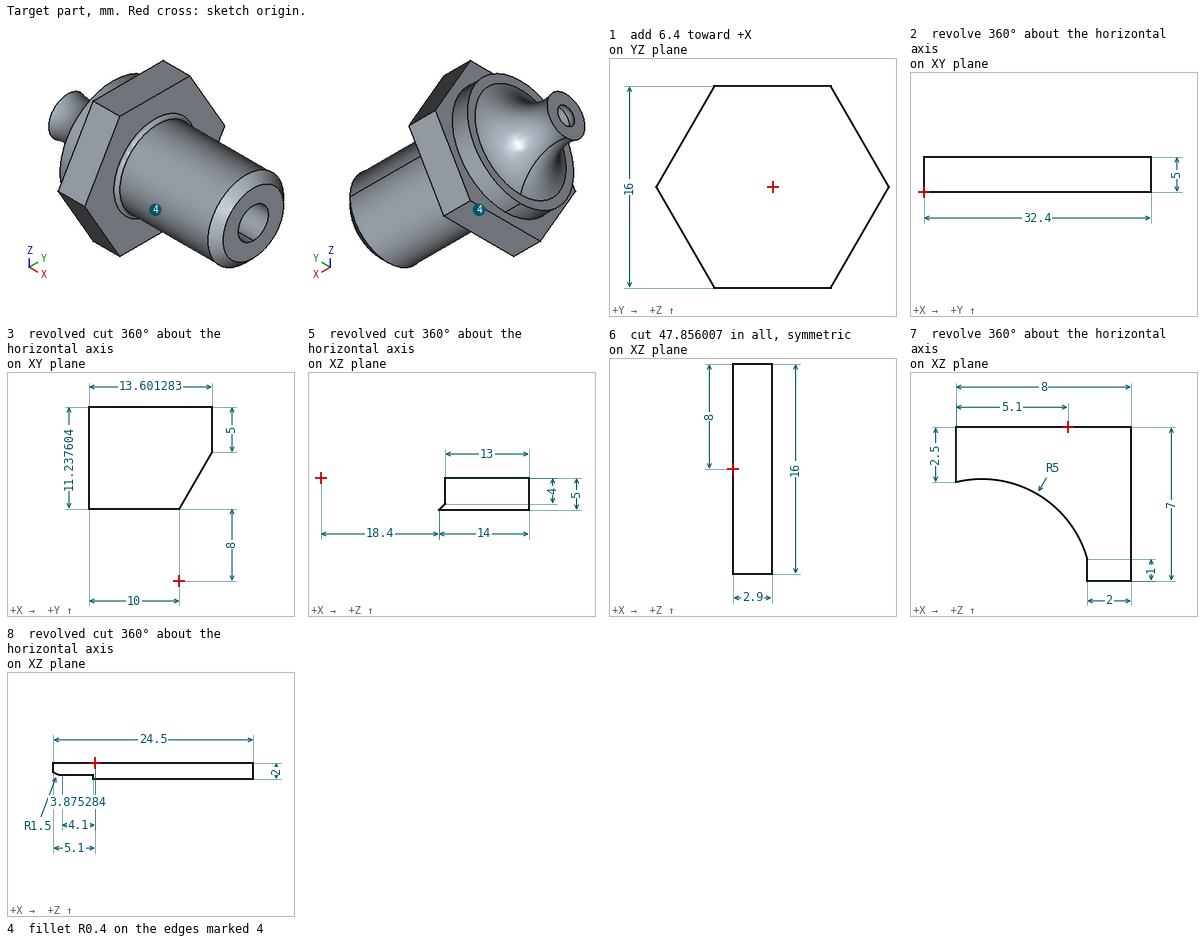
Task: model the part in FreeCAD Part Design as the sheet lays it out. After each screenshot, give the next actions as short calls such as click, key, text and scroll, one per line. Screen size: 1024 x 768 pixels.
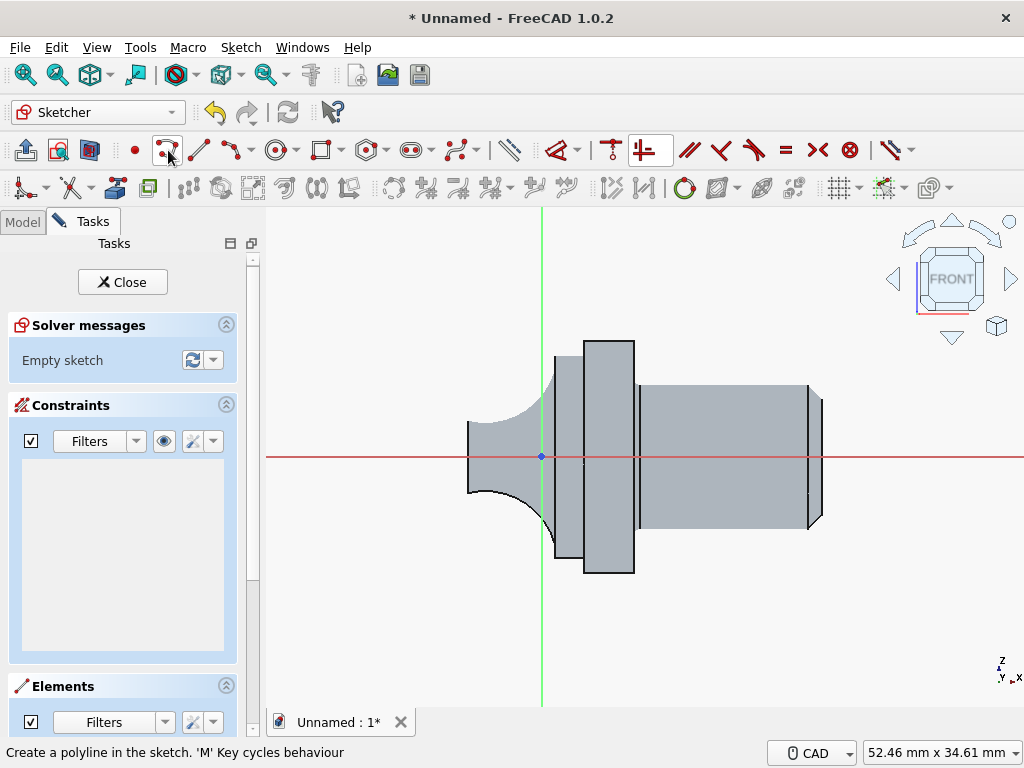
click(468, 473)
click(468, 457)
click(822, 466)
click(822, 486)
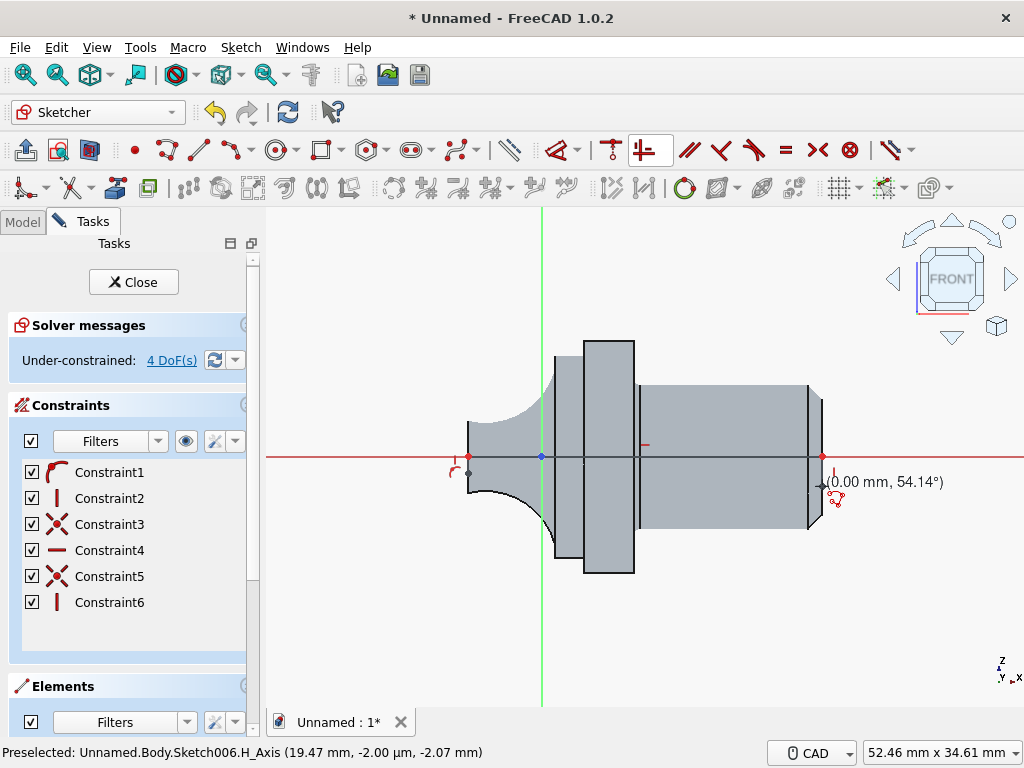
scroll(538, 486, up, 8)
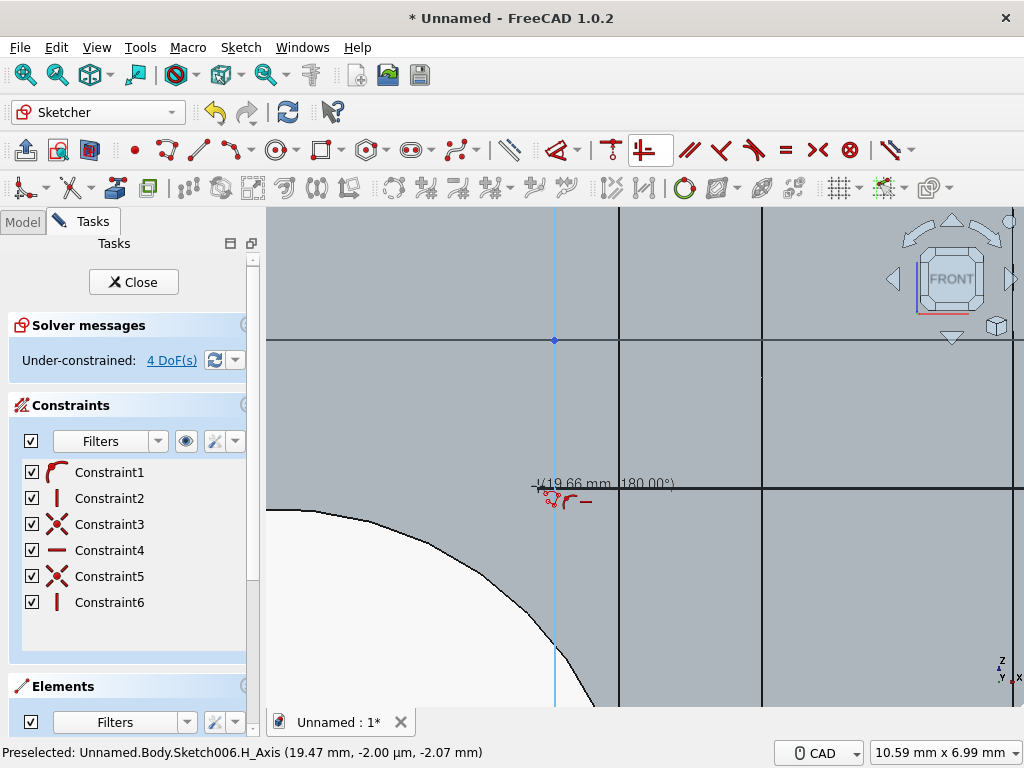
click(539, 484)
click(539, 447)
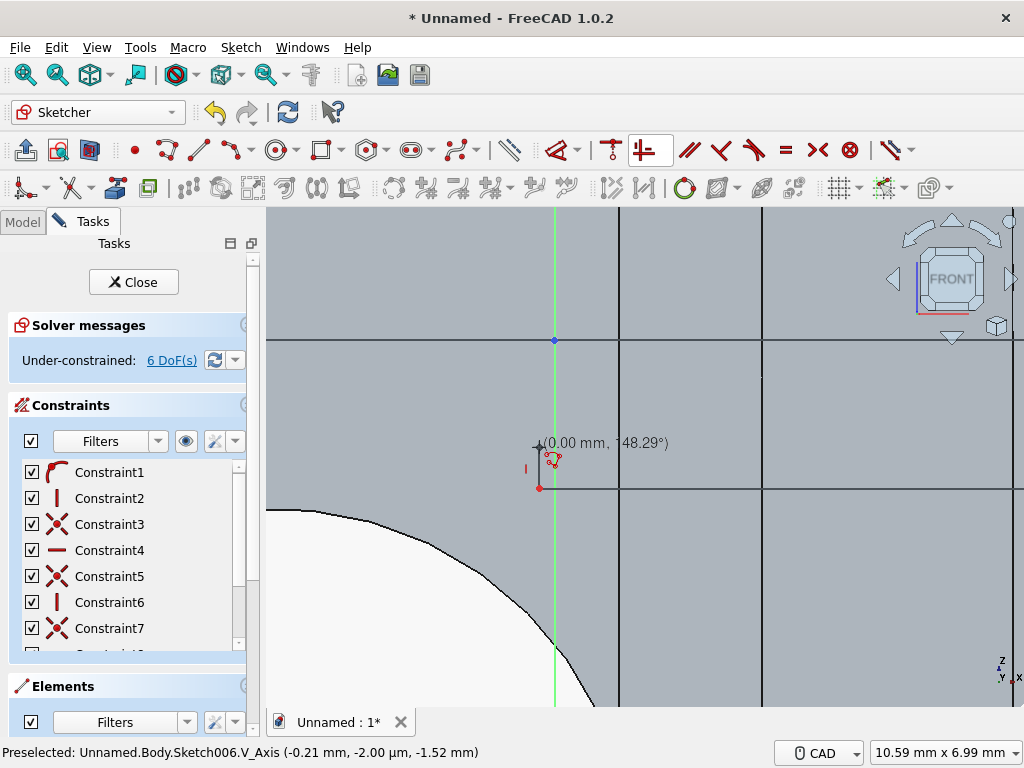
scroll(416, 472, down, 7)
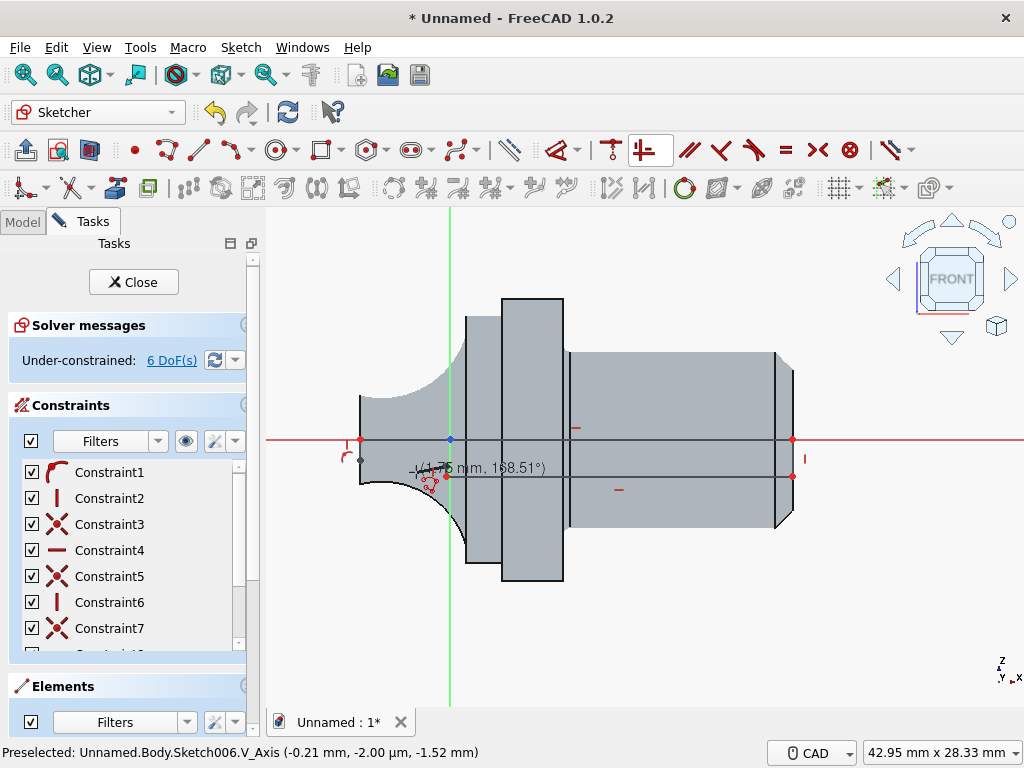
click(378, 466)
right_click(378, 466)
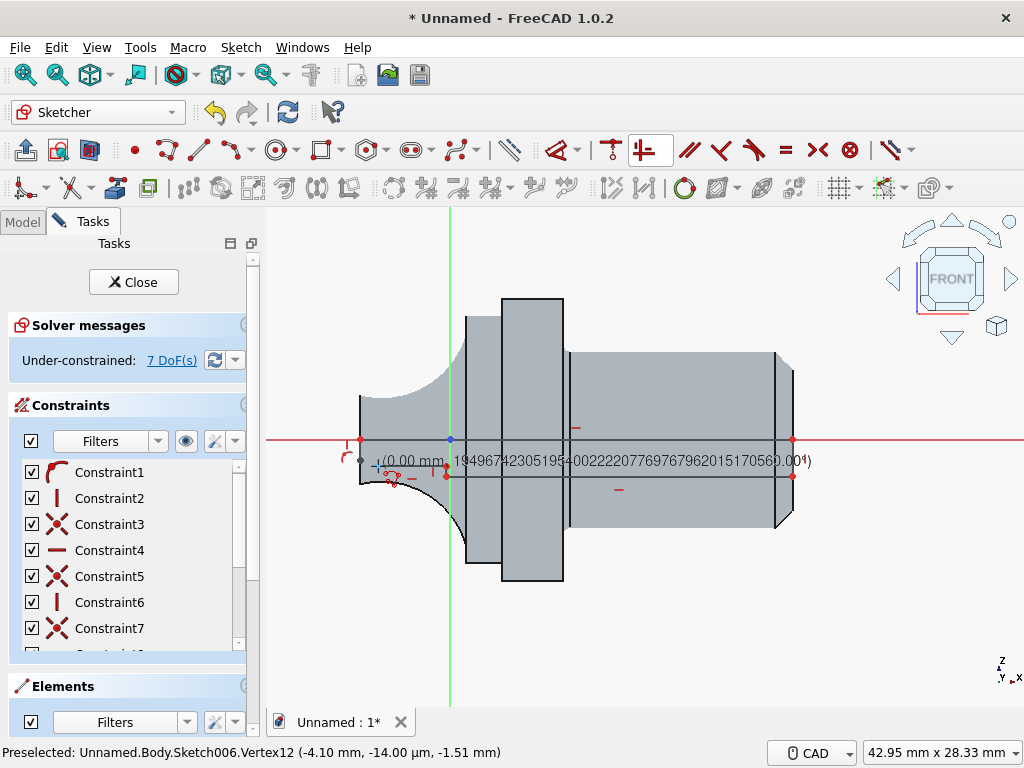
click(232, 150)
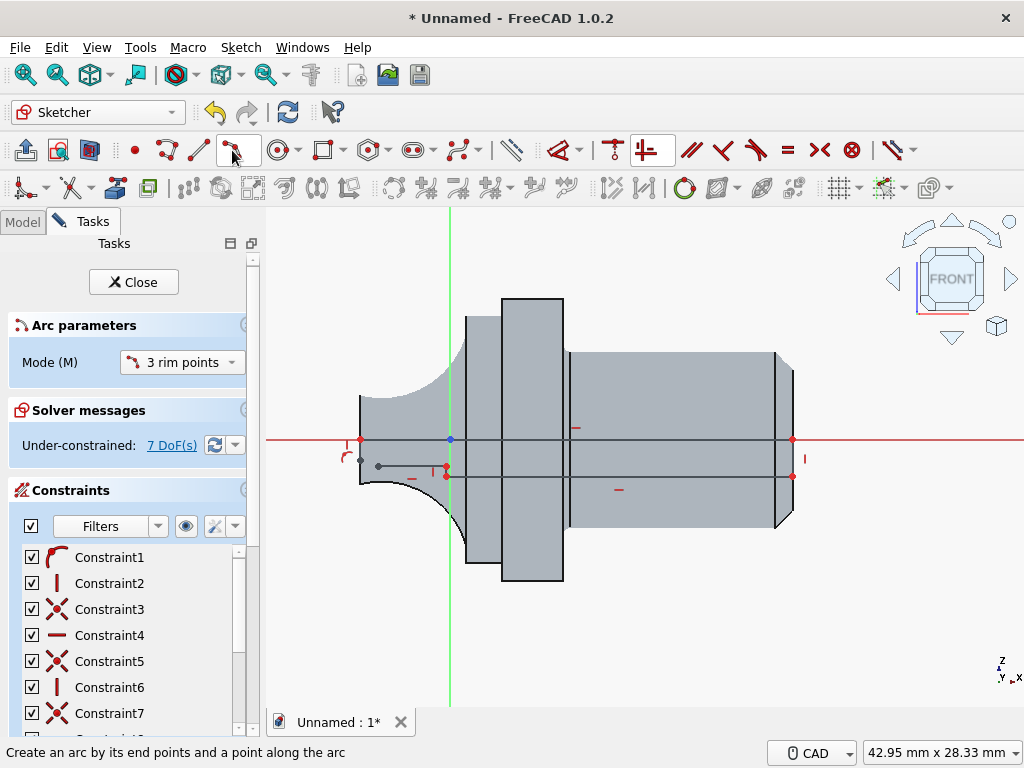
click(378, 466)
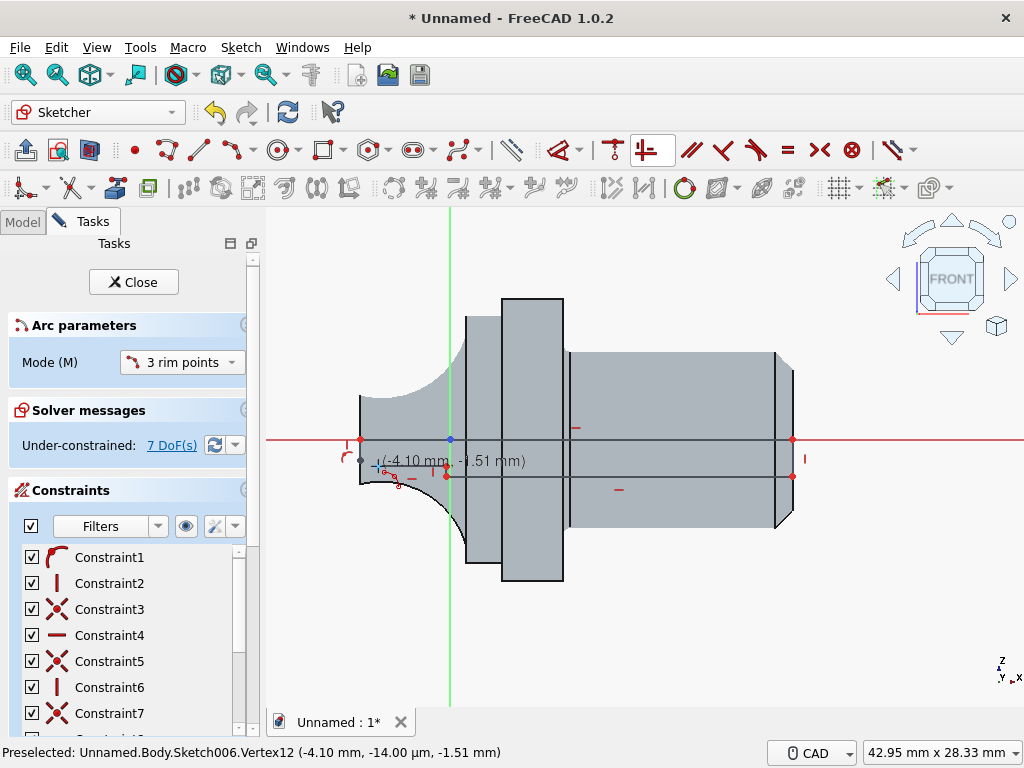
scroll(360, 460, up, 3)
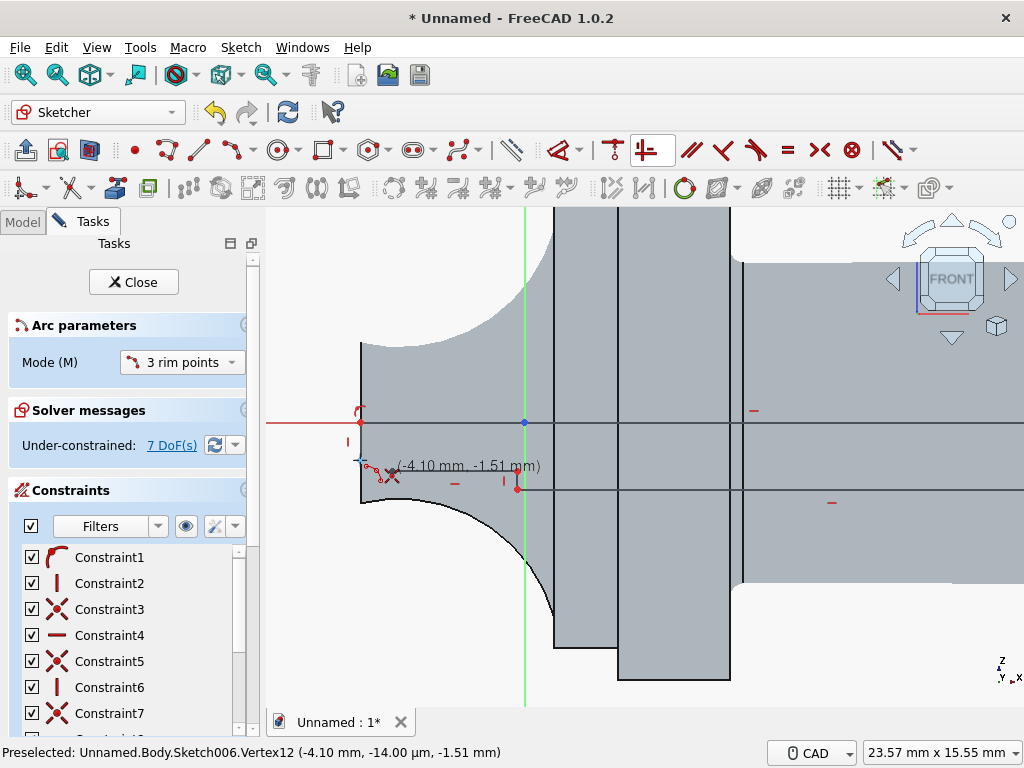
click(361, 461)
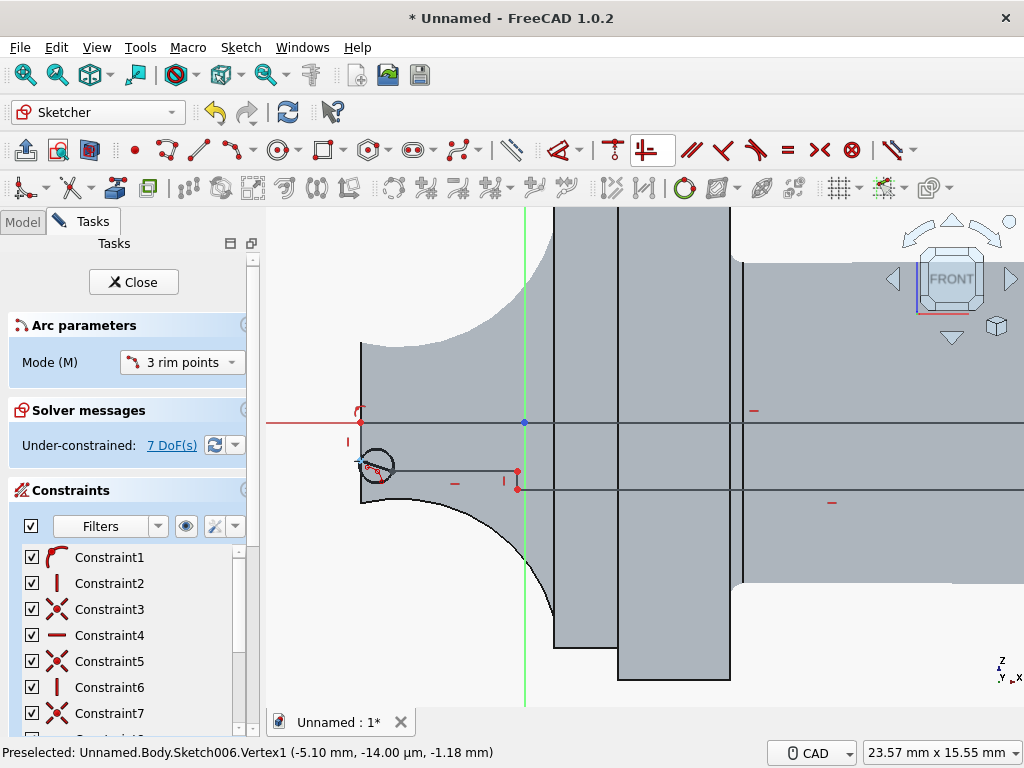
scroll(376, 468, up, 9)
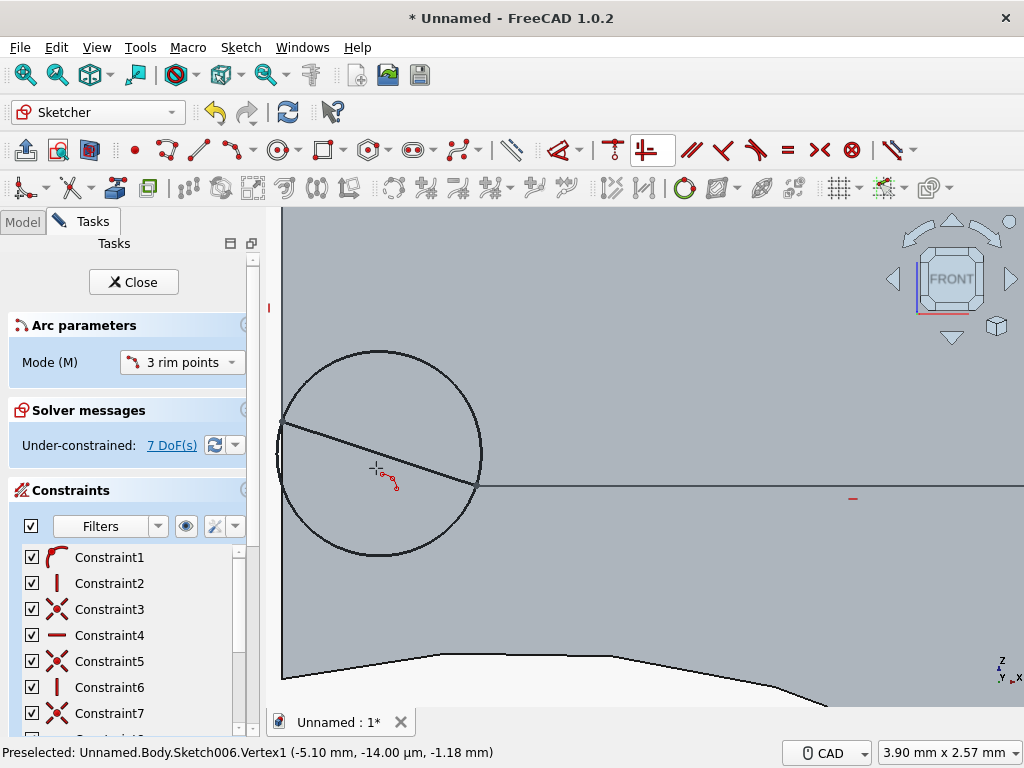
click(373, 465)
key(Escape)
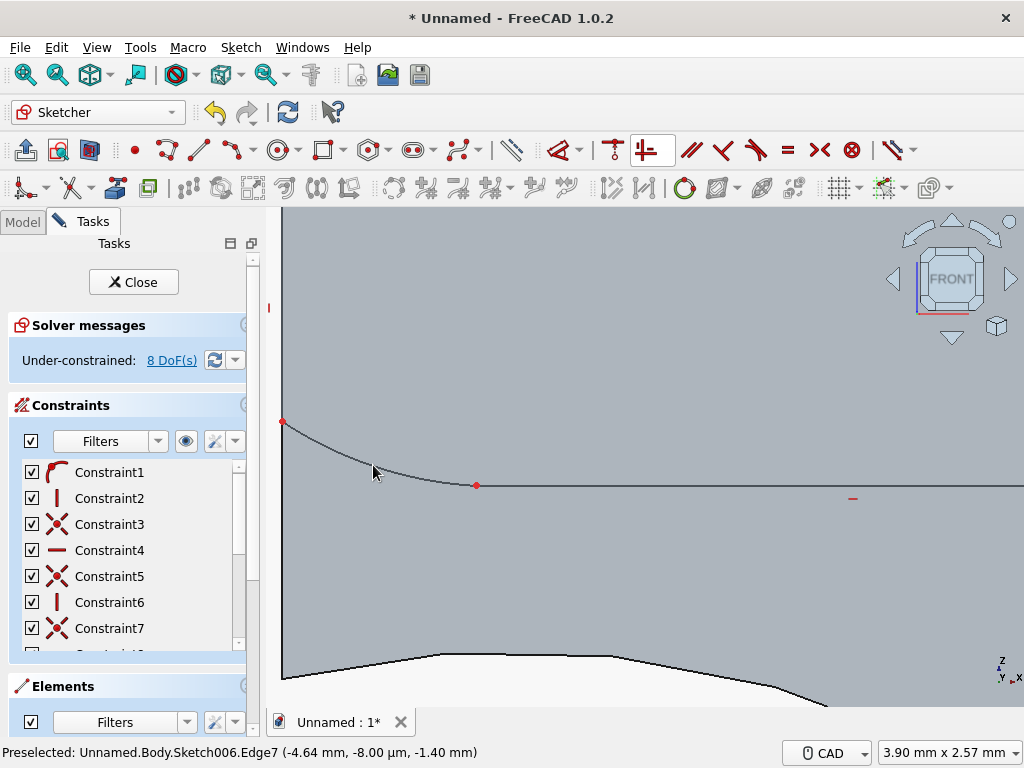
scroll(368, 464, down, 12)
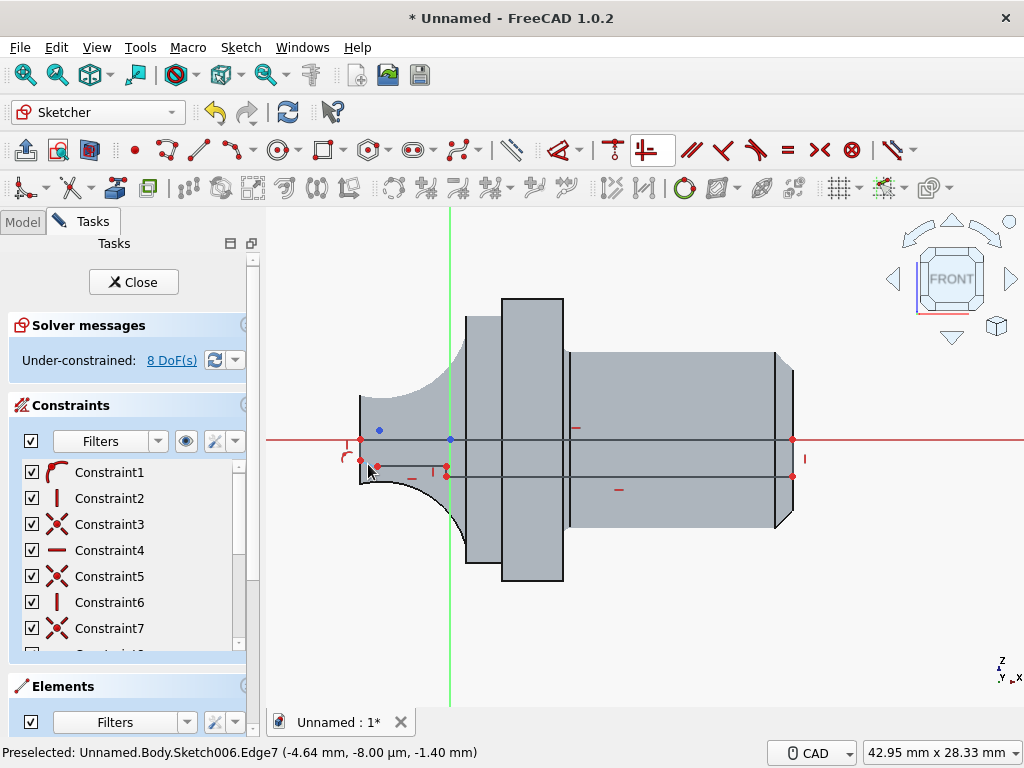
click(398, 466)